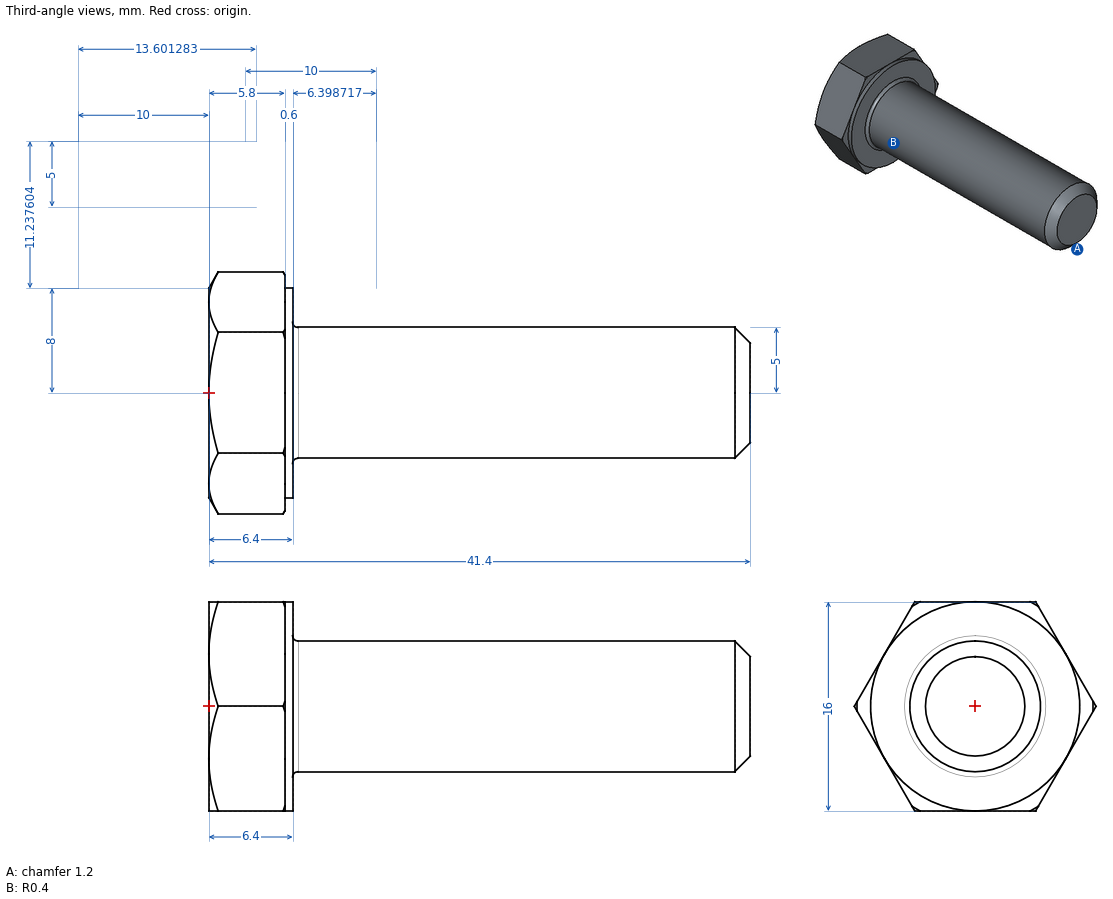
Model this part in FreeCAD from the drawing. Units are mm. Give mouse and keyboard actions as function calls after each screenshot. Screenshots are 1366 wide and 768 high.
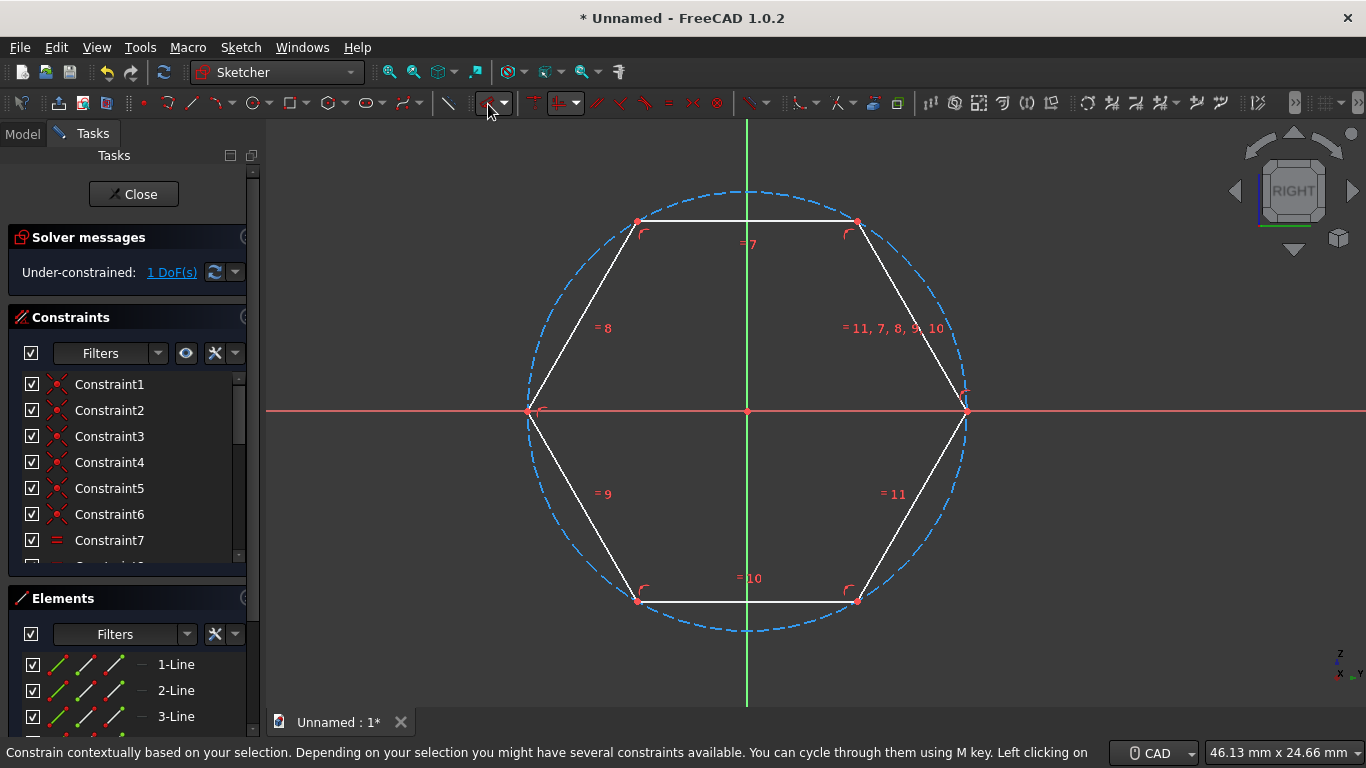
click(637, 602)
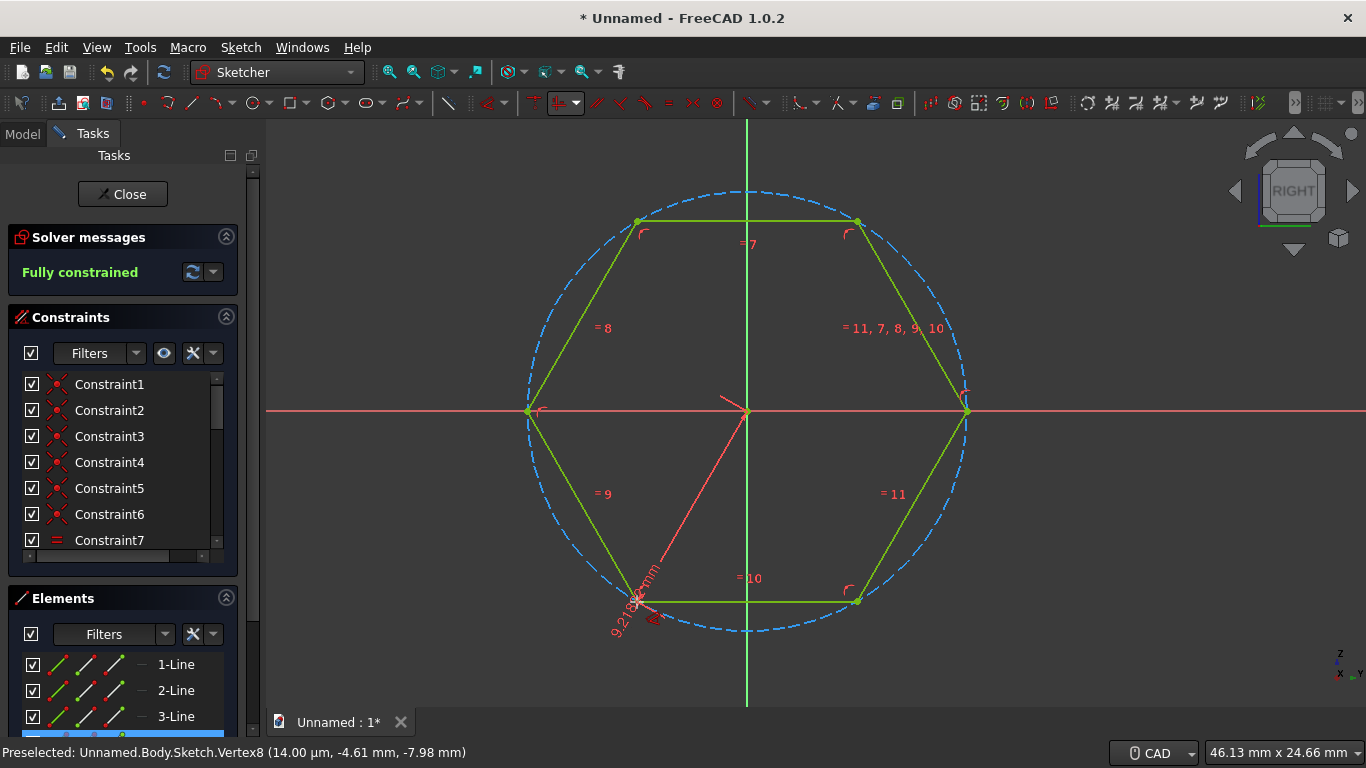
click(857, 221)
click(891, 324)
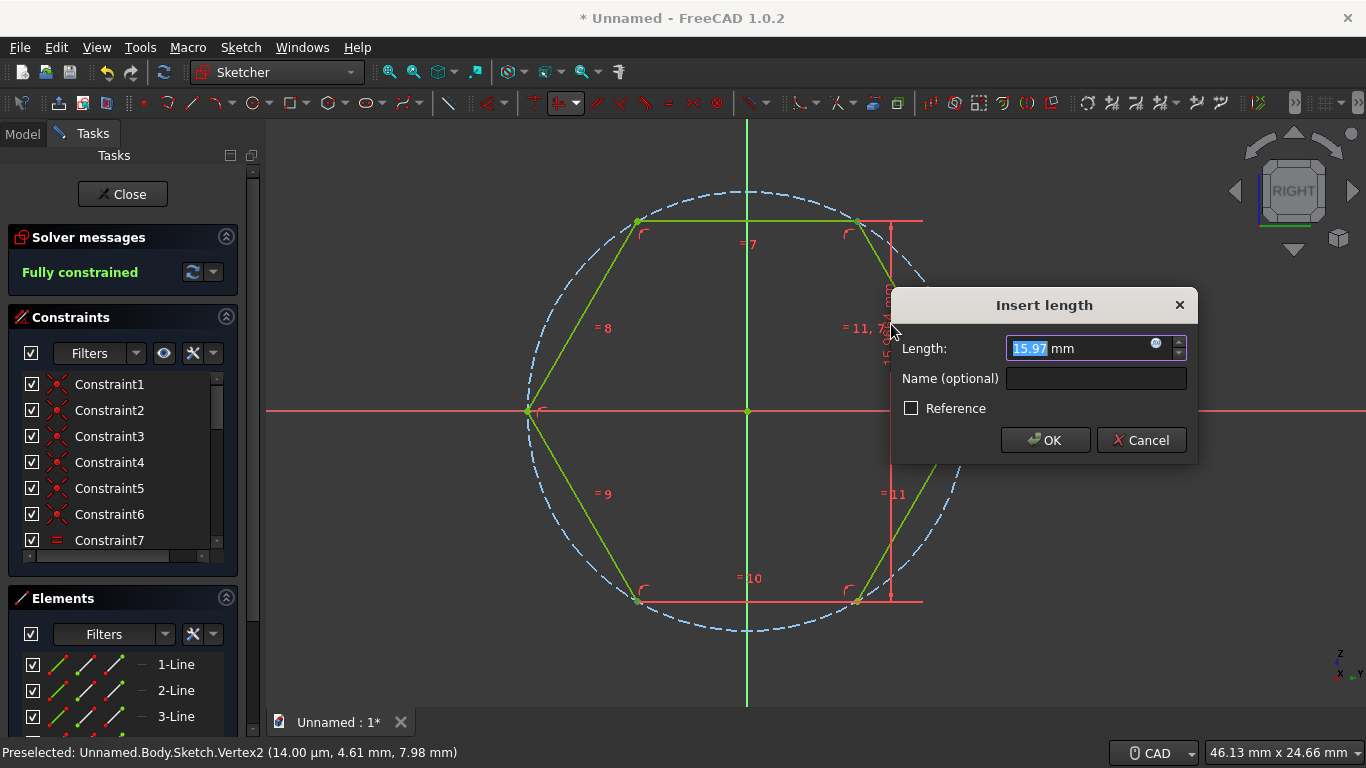
text(16)
key(Return)
key(Escape)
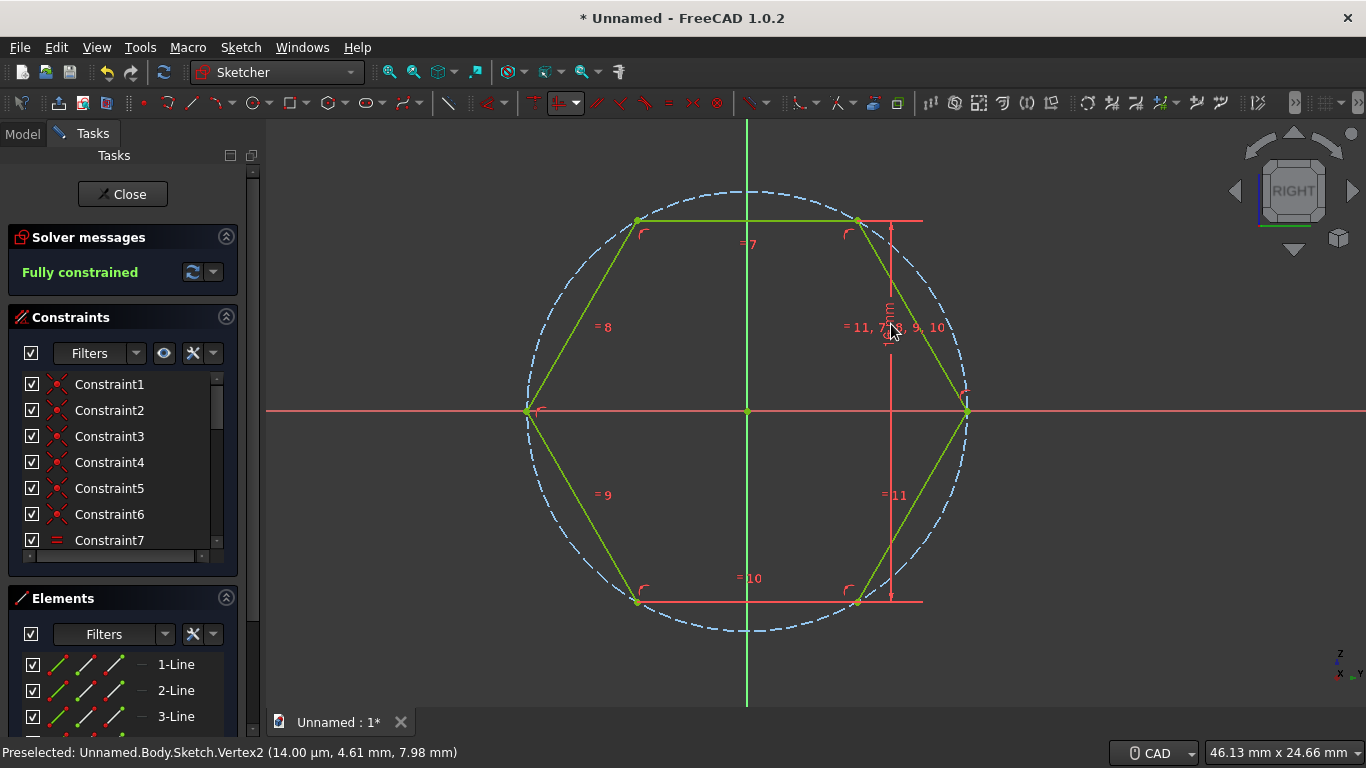
click(123, 194)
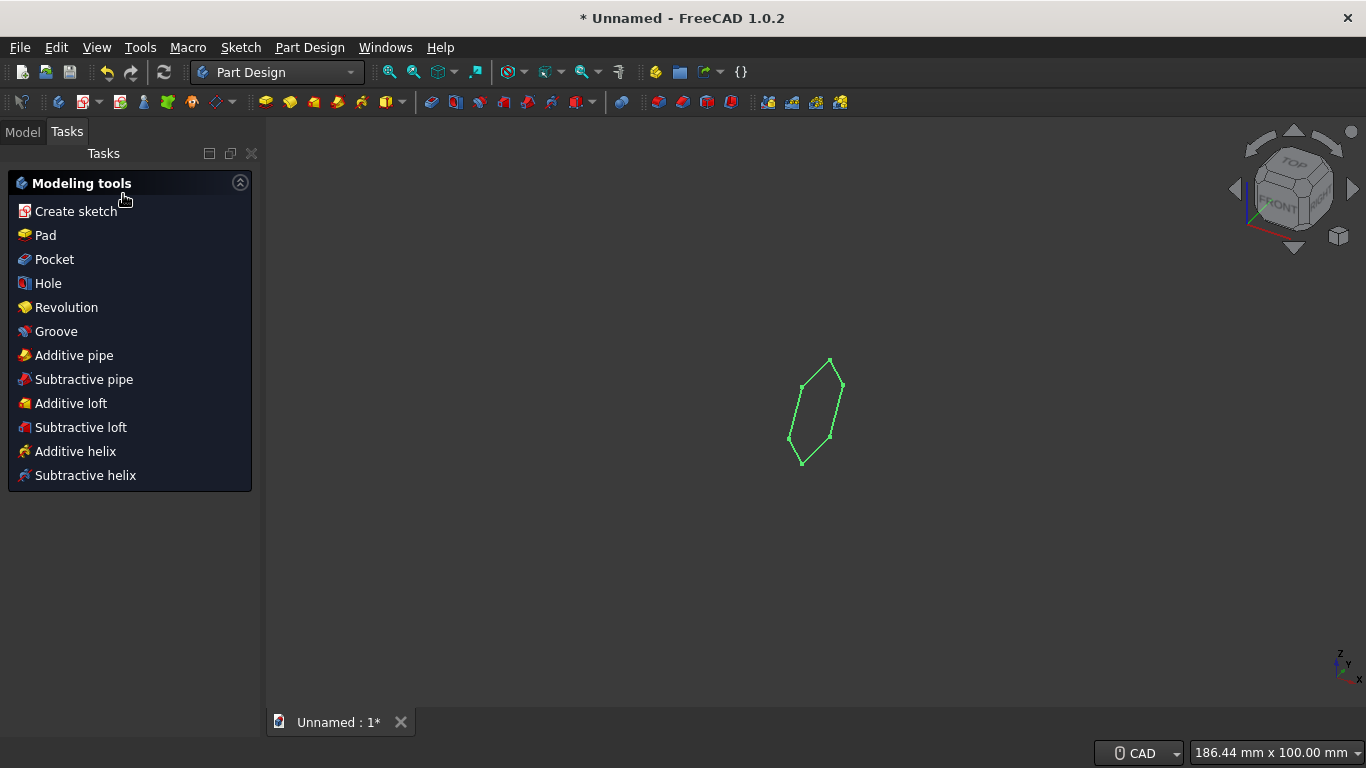
click(266, 102)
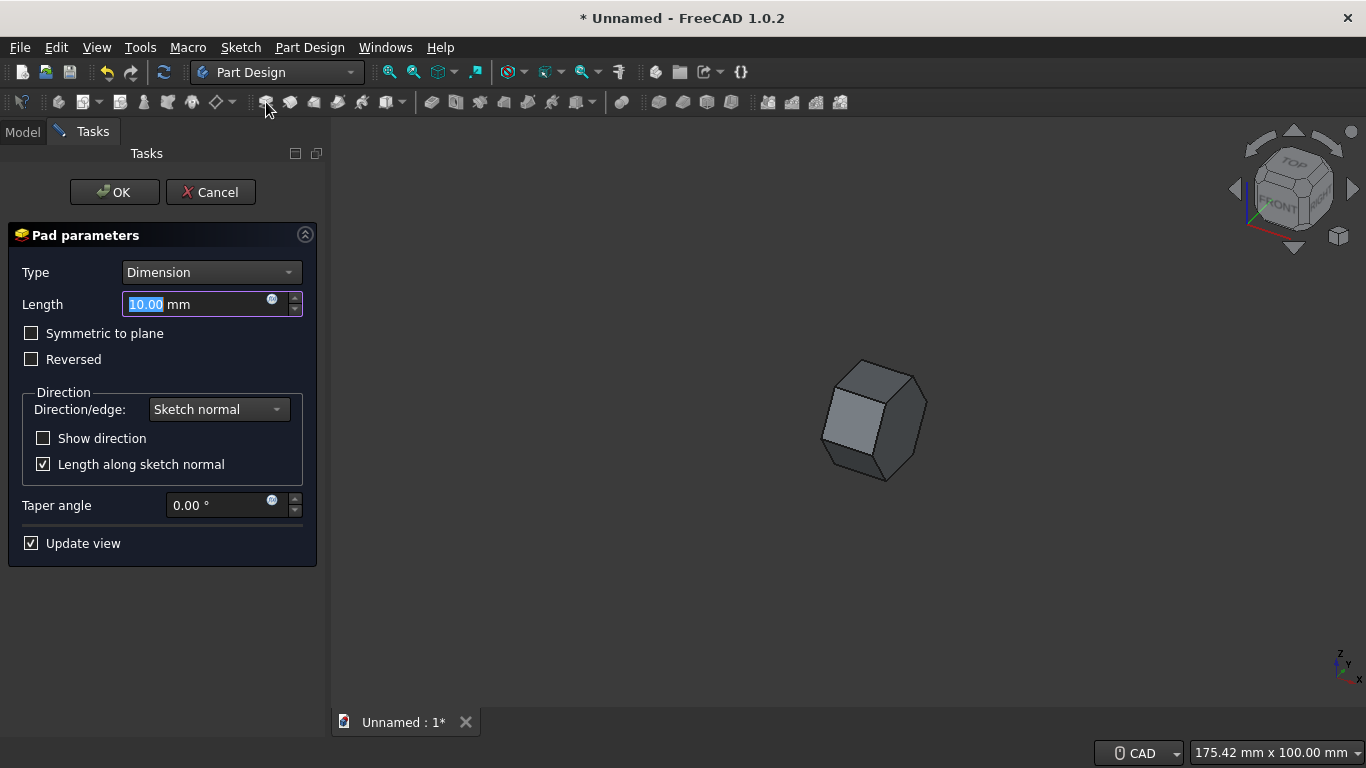
text(6.4)
key(Tab)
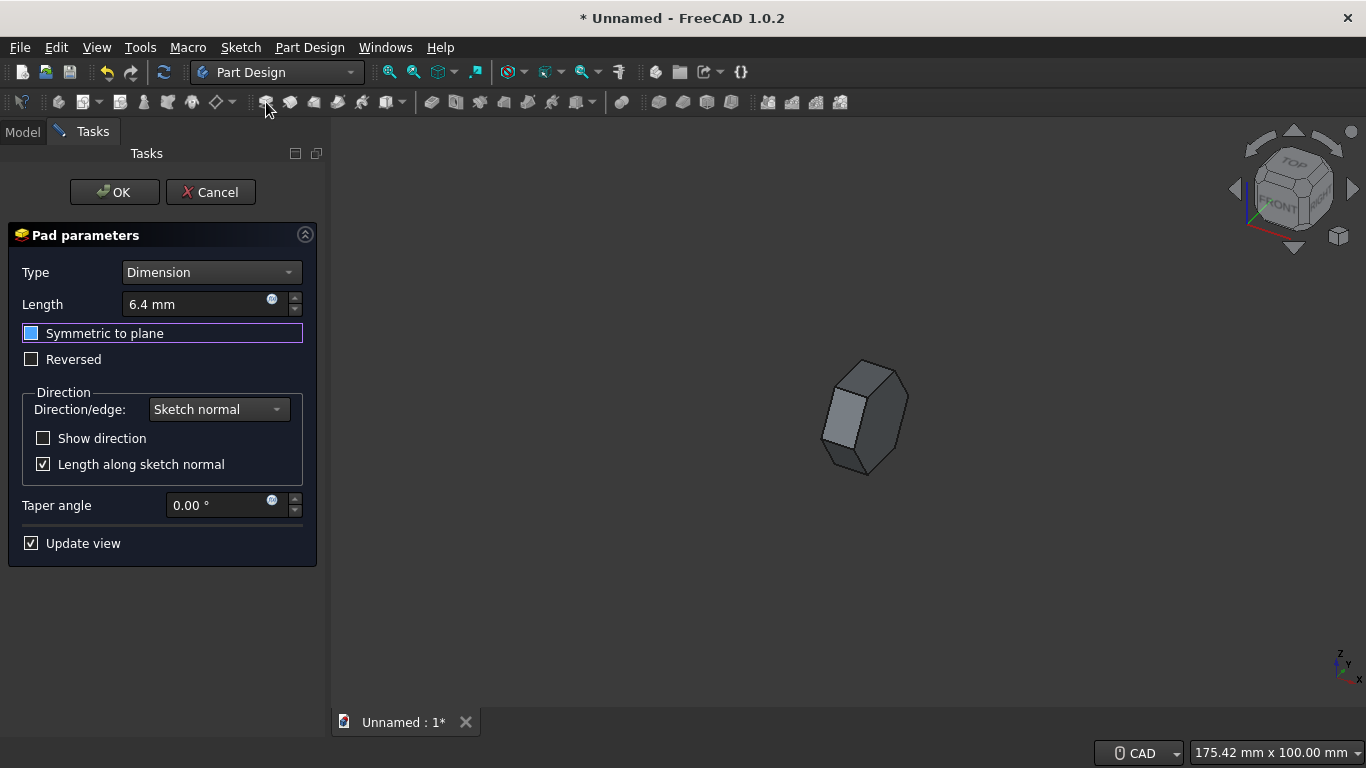
click(115, 192)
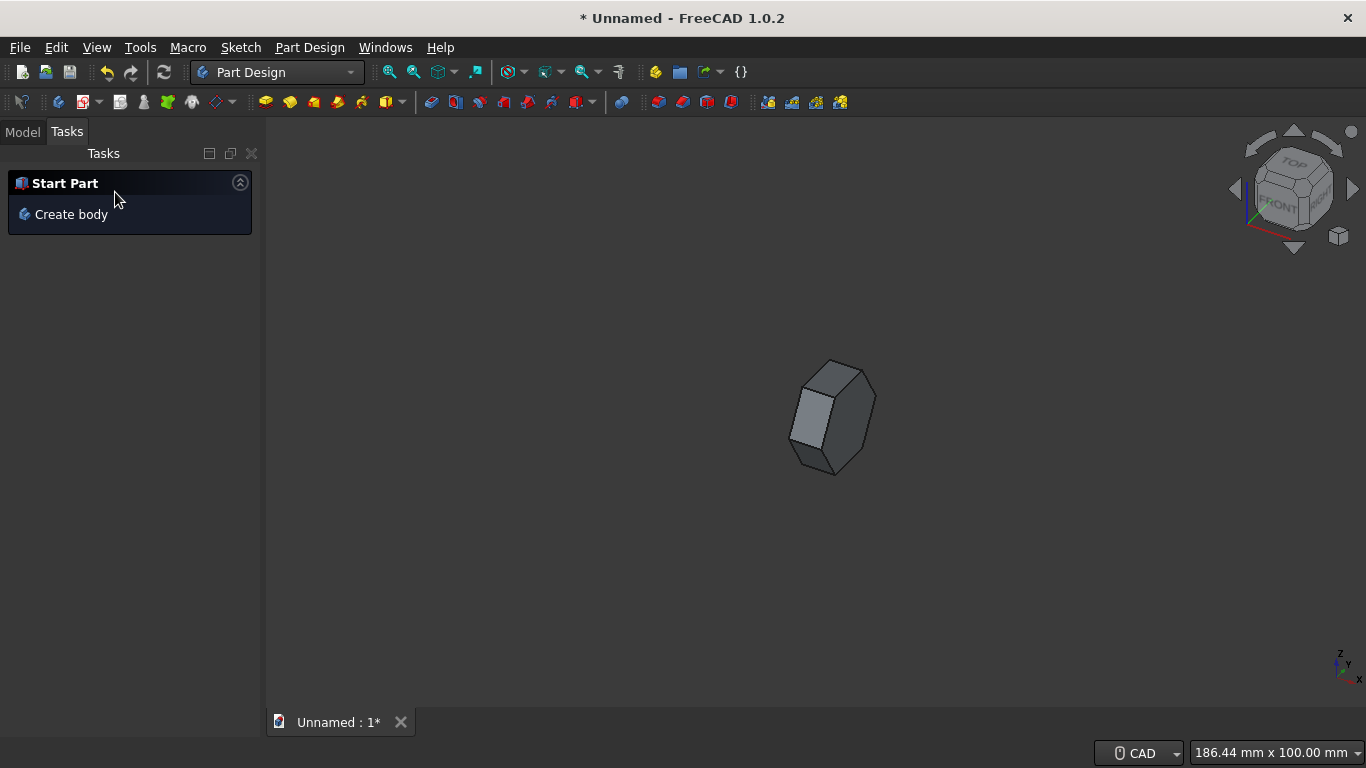
click(390, 72)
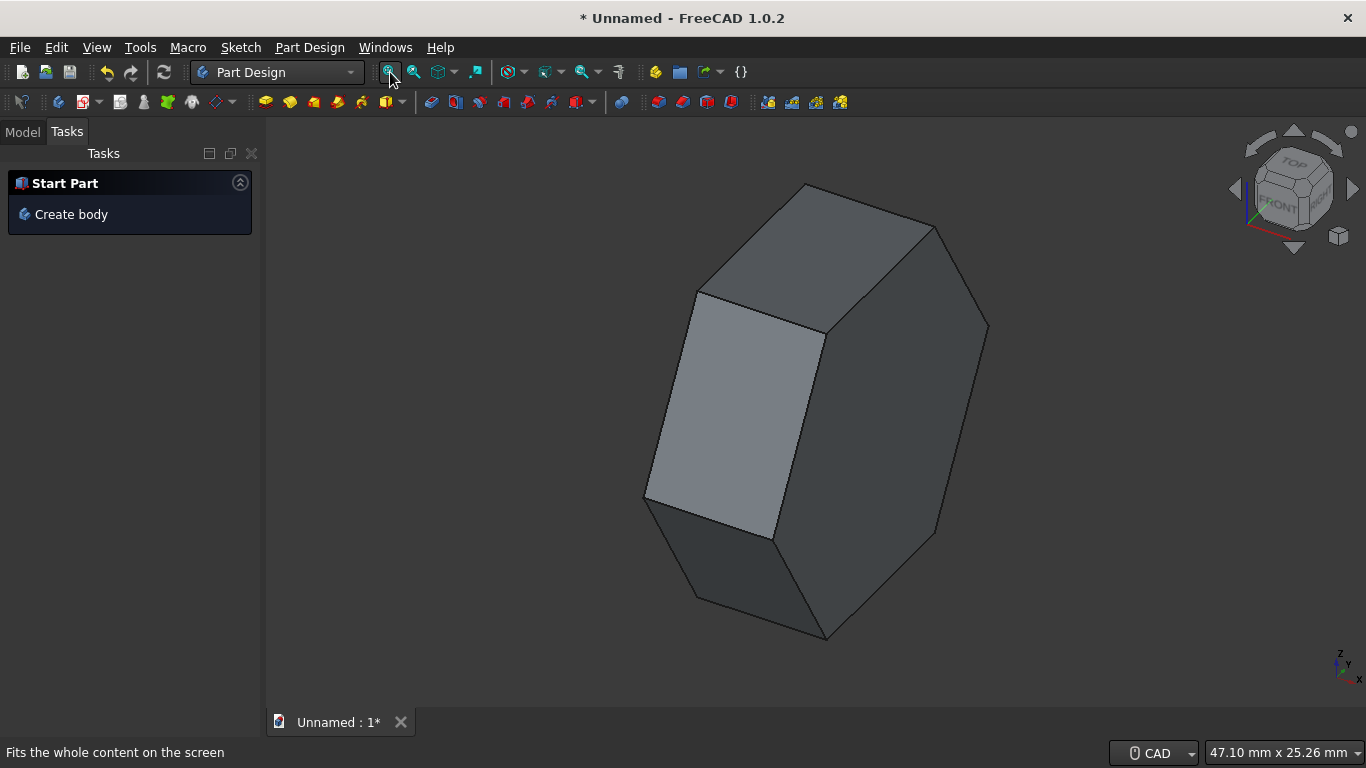
click(84, 102)